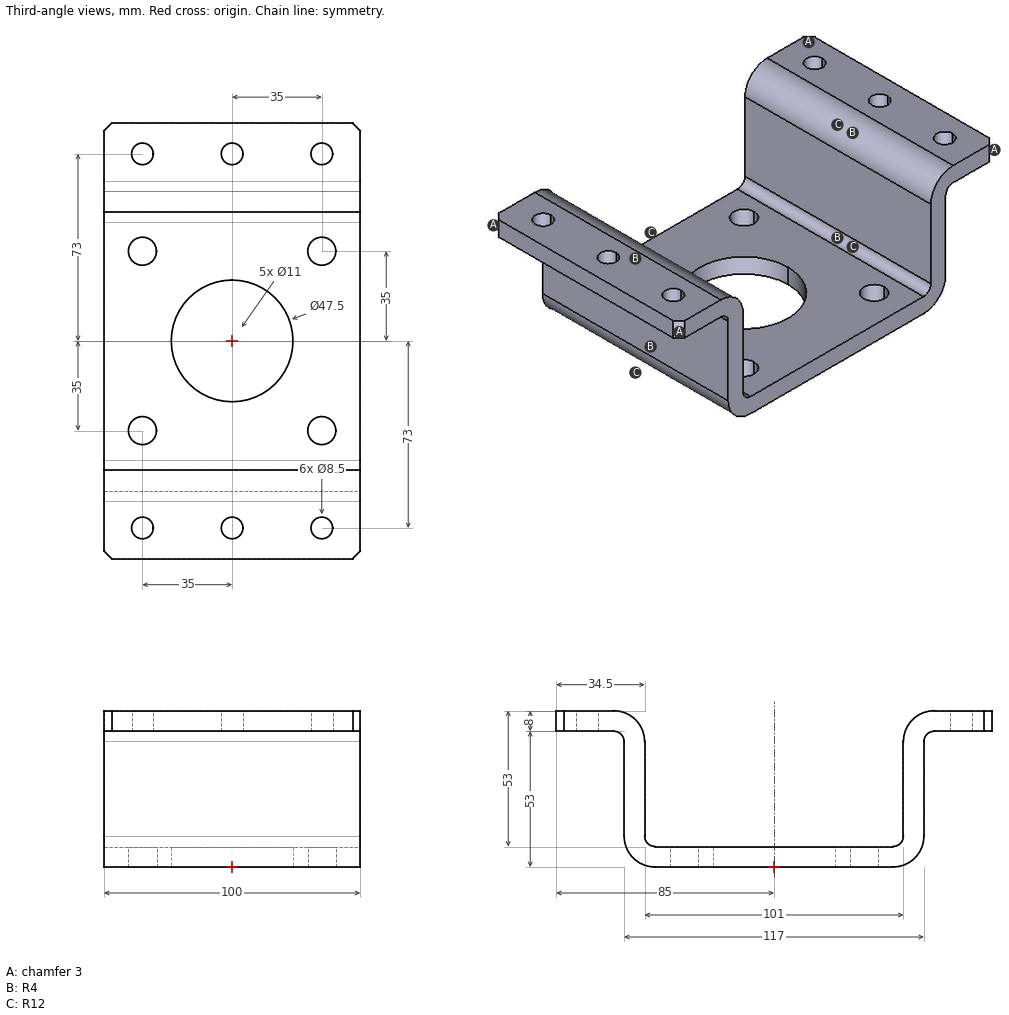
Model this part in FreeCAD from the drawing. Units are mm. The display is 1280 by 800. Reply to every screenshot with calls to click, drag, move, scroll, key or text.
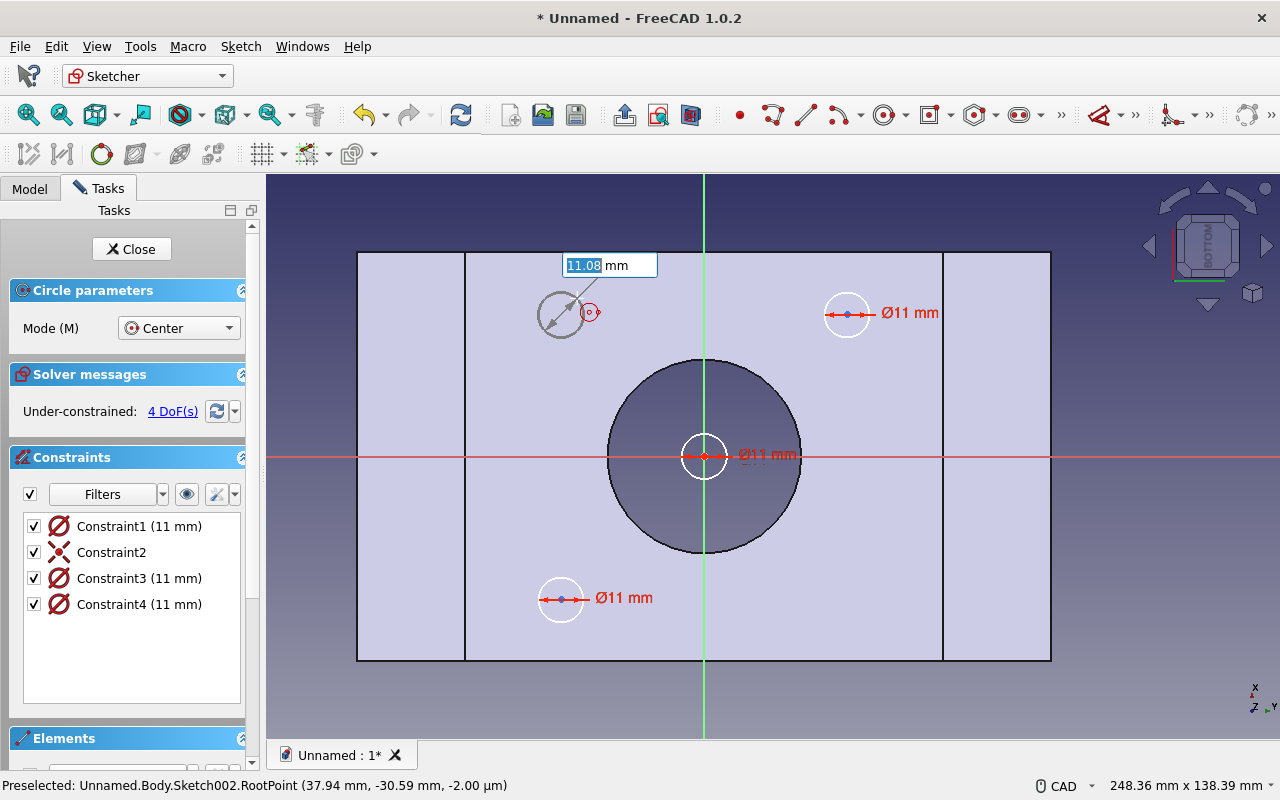
text(11)
key(Return)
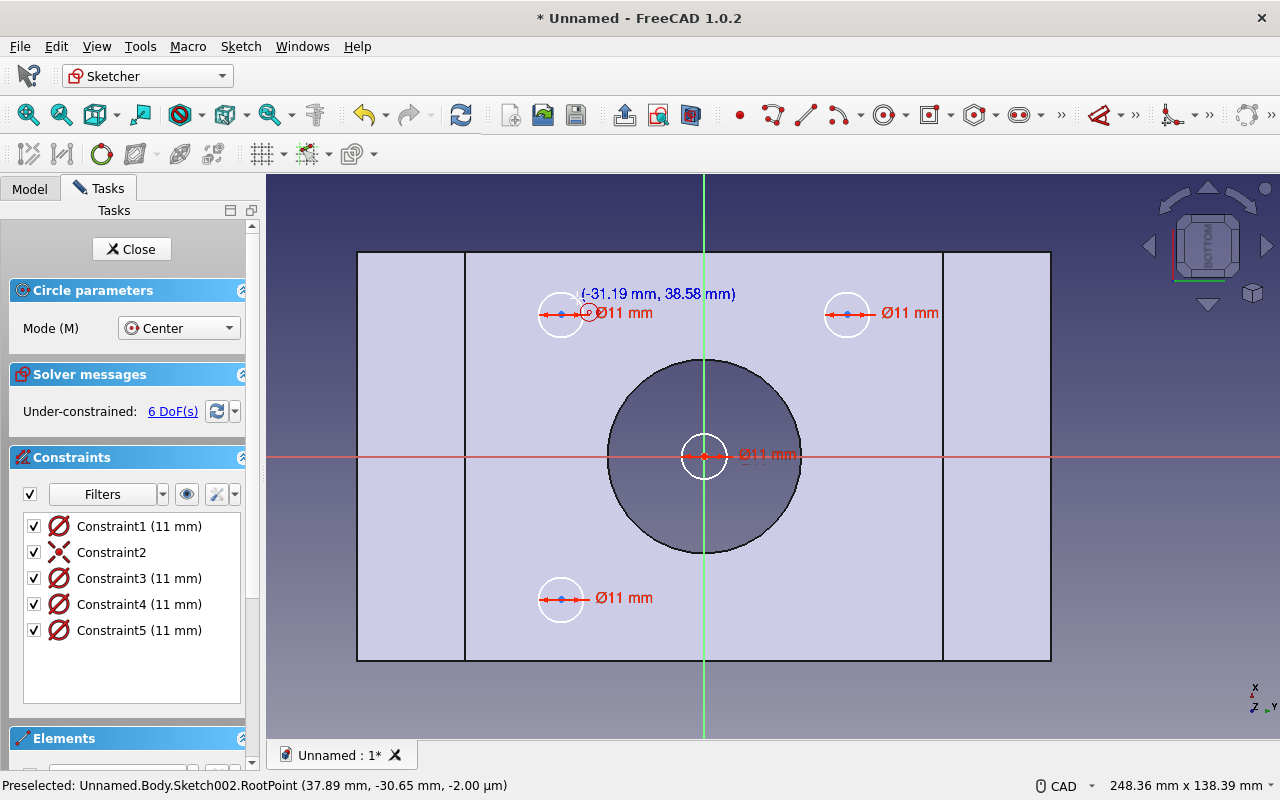
click(847, 599)
move(863, 584)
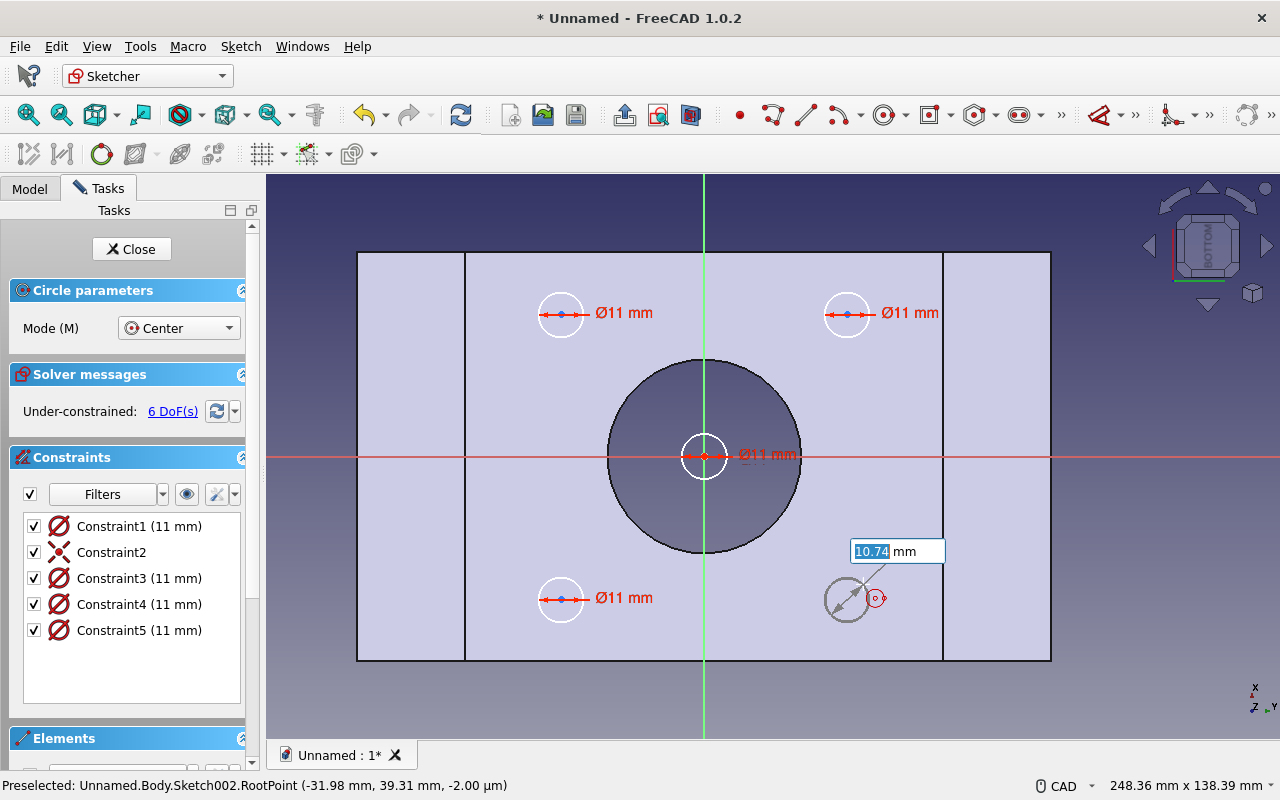
text(11)
key(Return)
key(Escape)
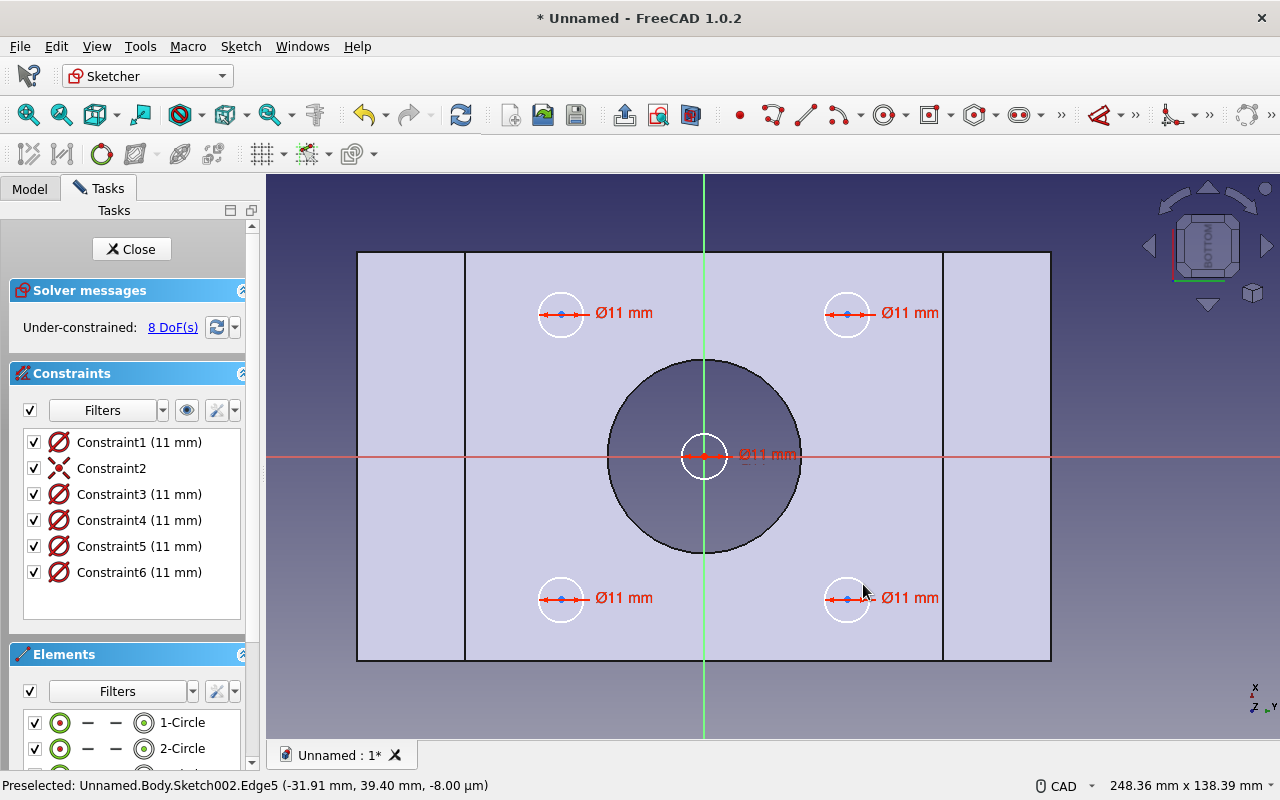
click(561, 600)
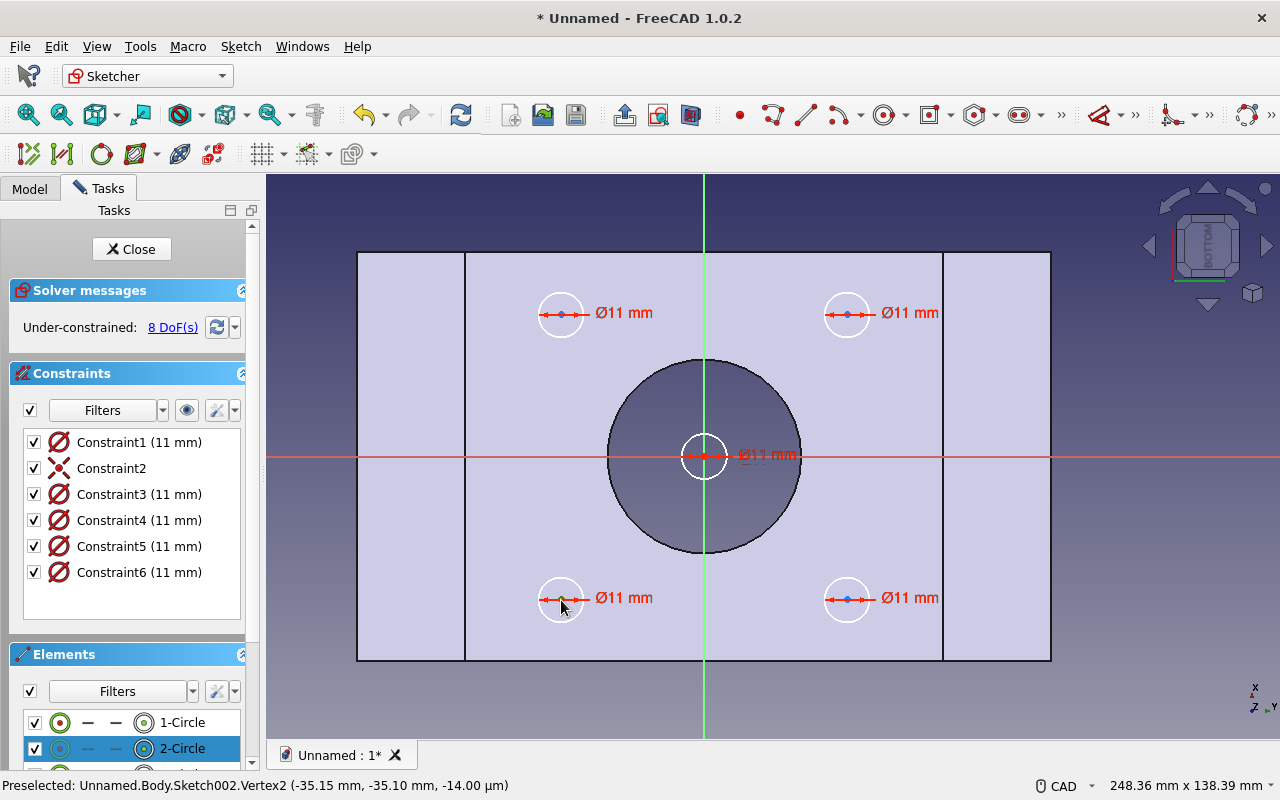
click(561, 315)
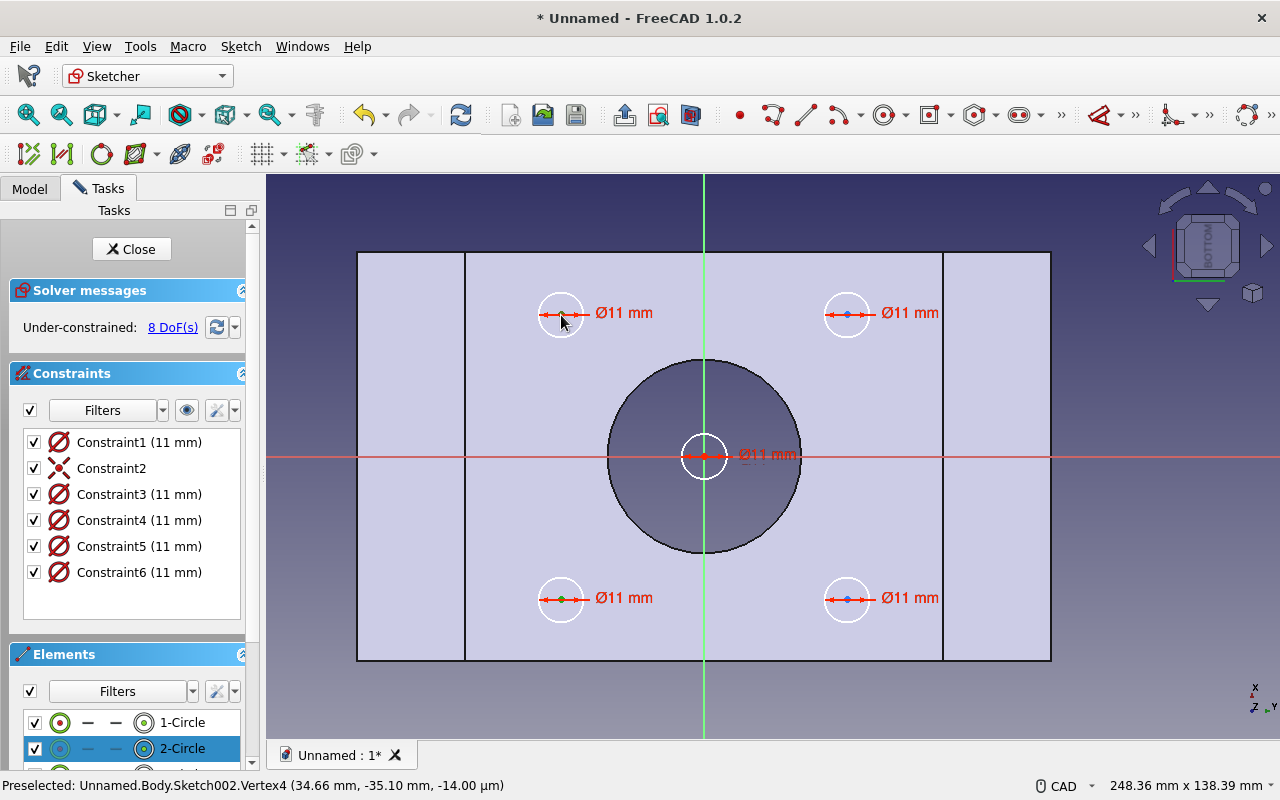
key(v)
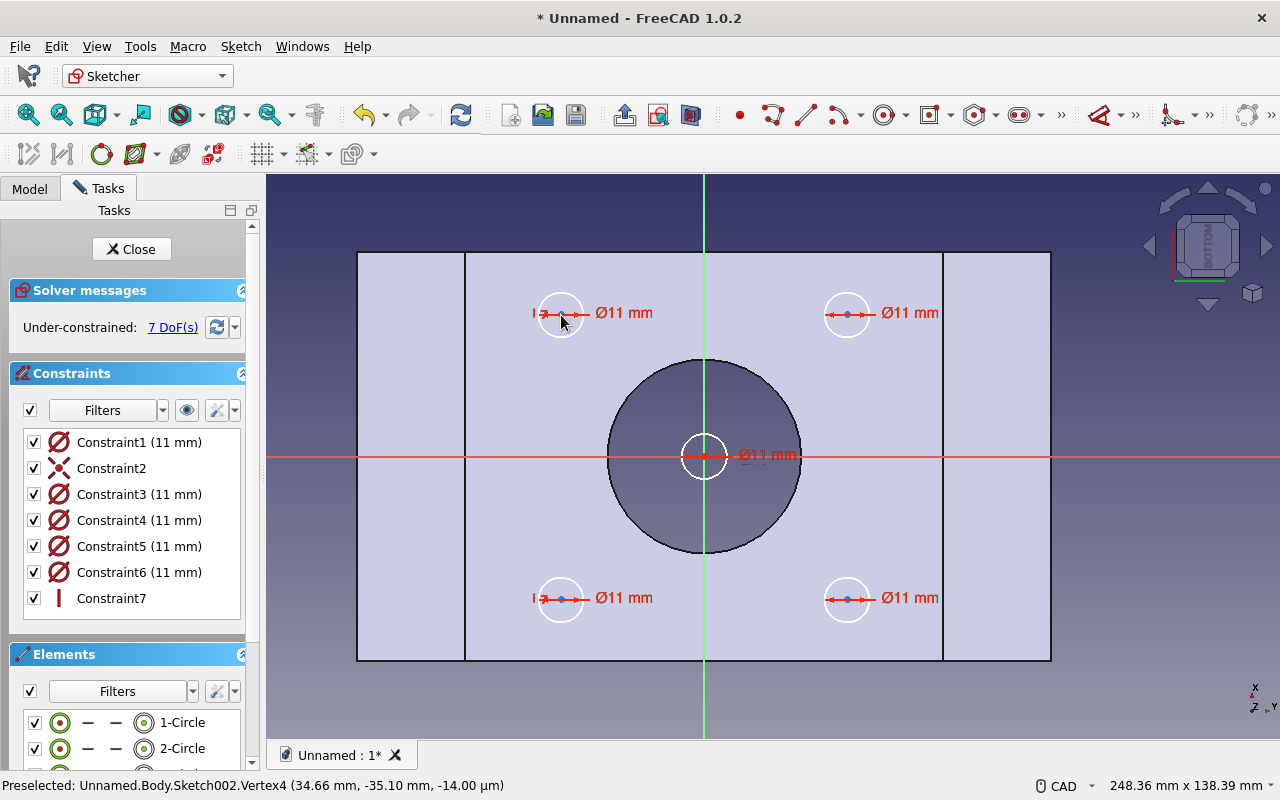
click(847, 315)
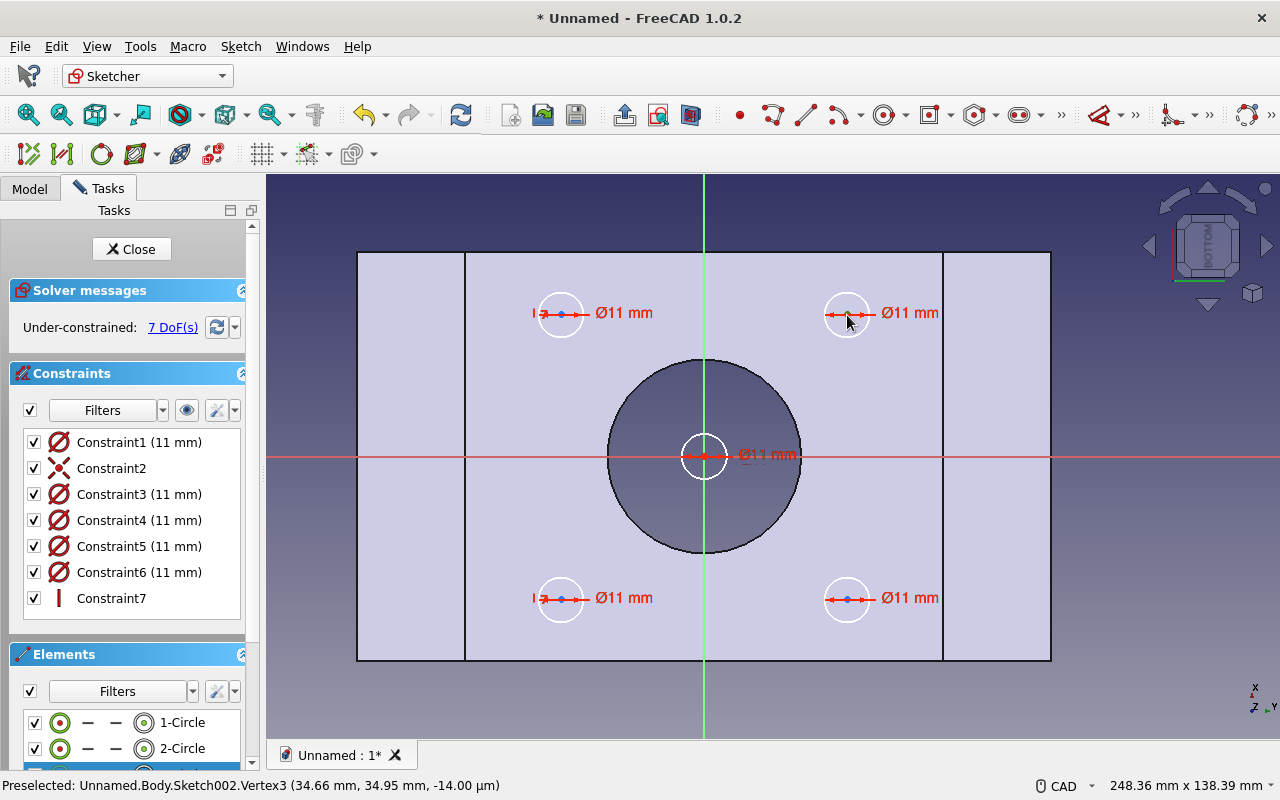
click(561, 315)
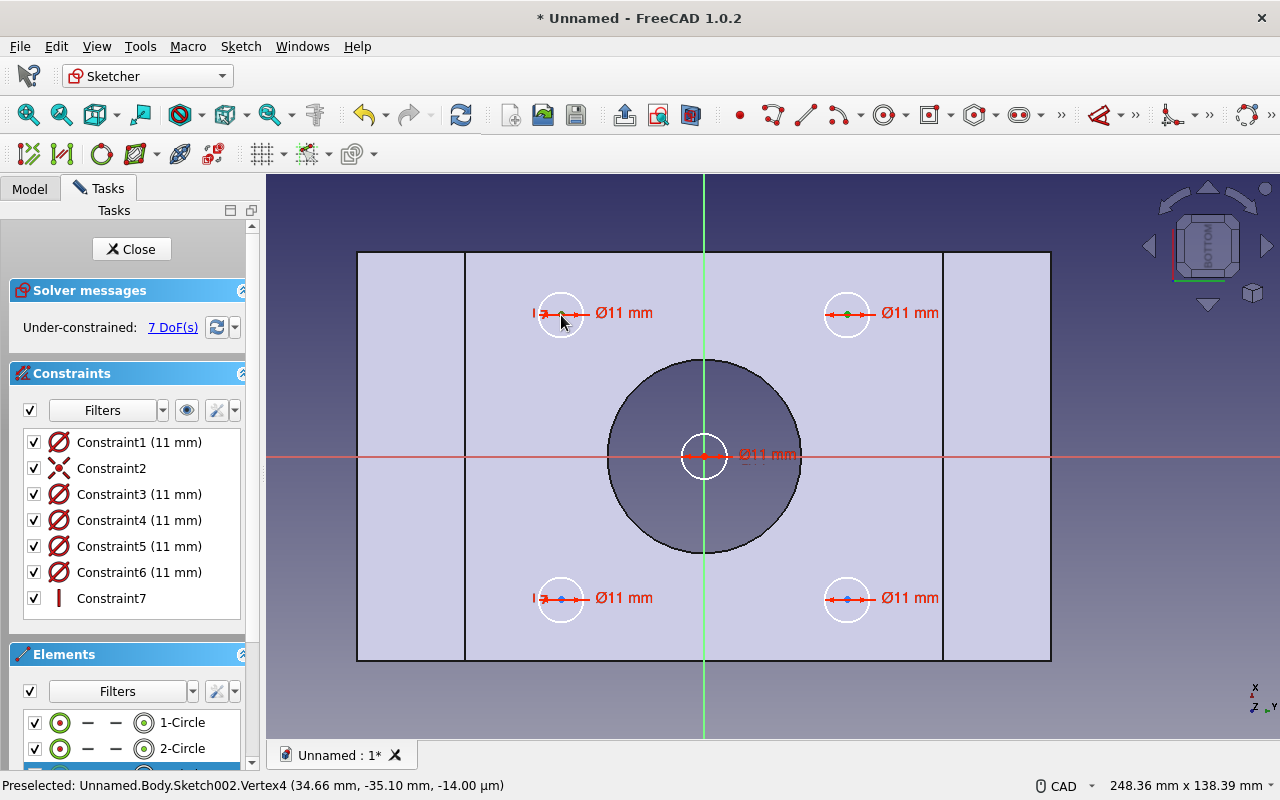
key(h)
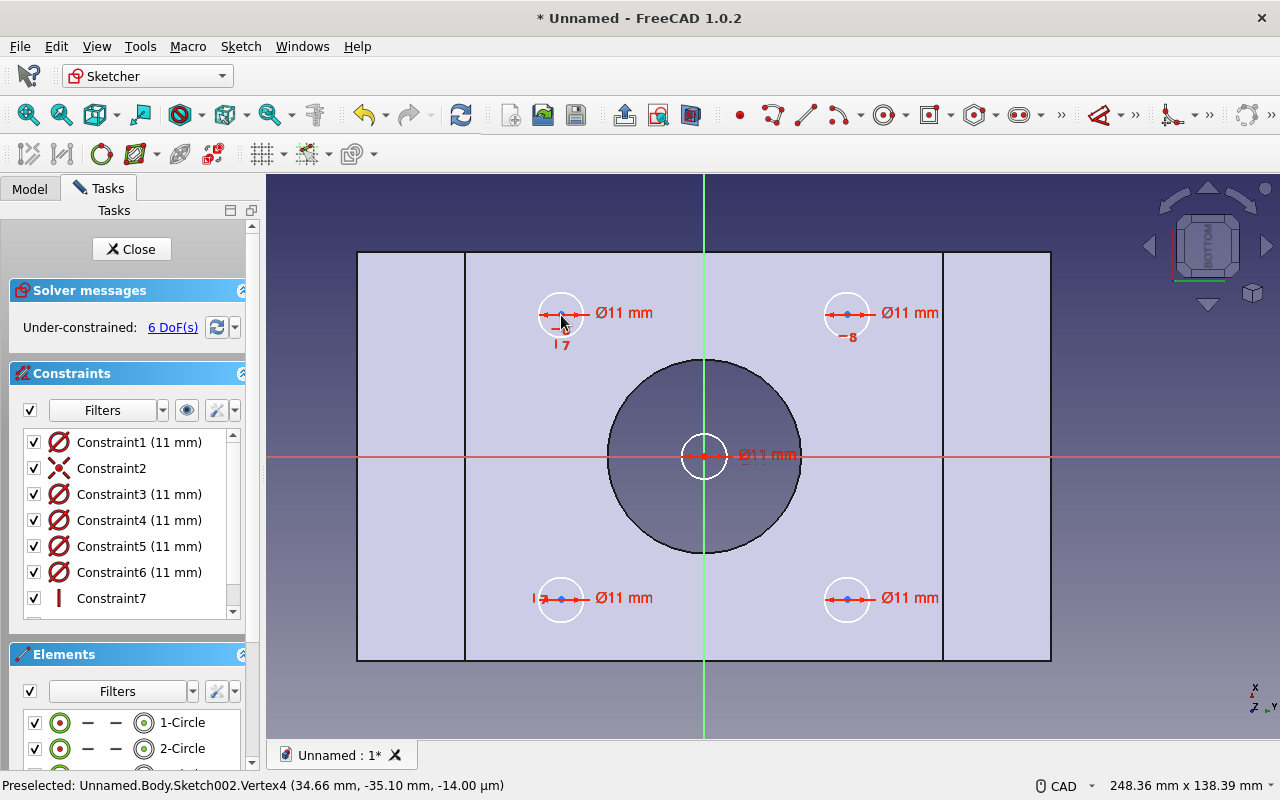
click(847, 315)